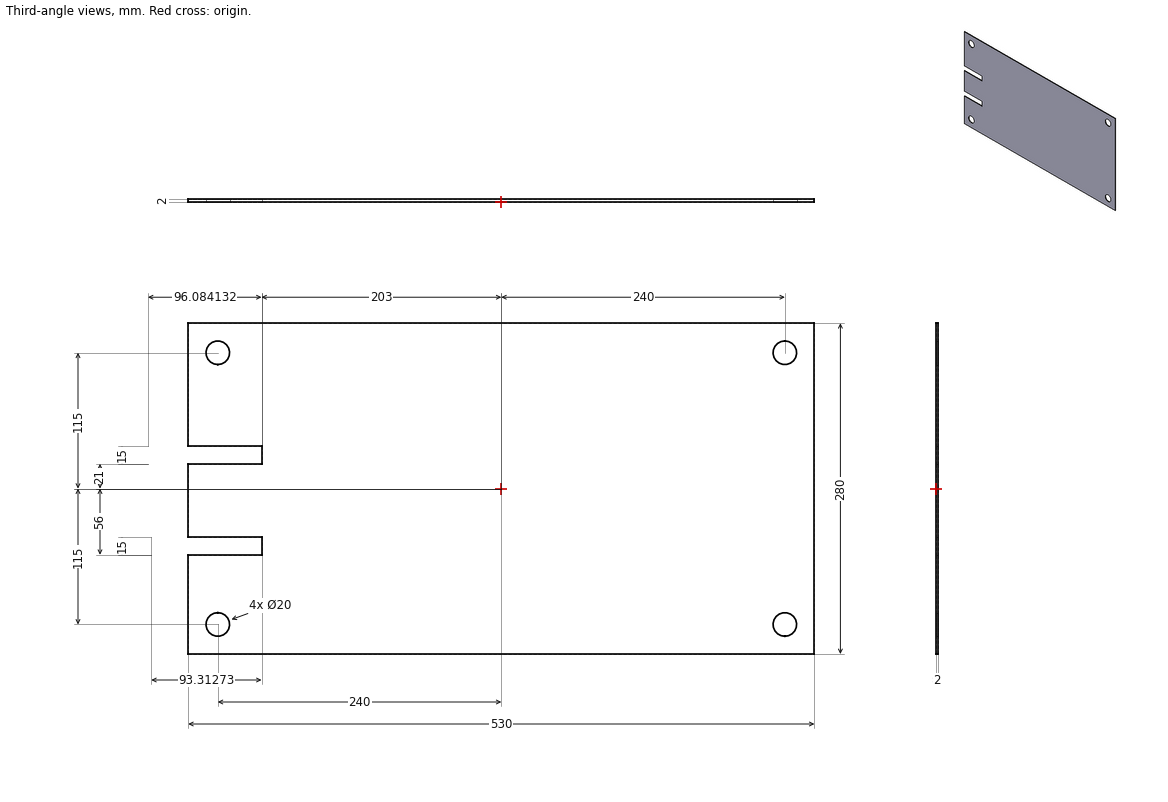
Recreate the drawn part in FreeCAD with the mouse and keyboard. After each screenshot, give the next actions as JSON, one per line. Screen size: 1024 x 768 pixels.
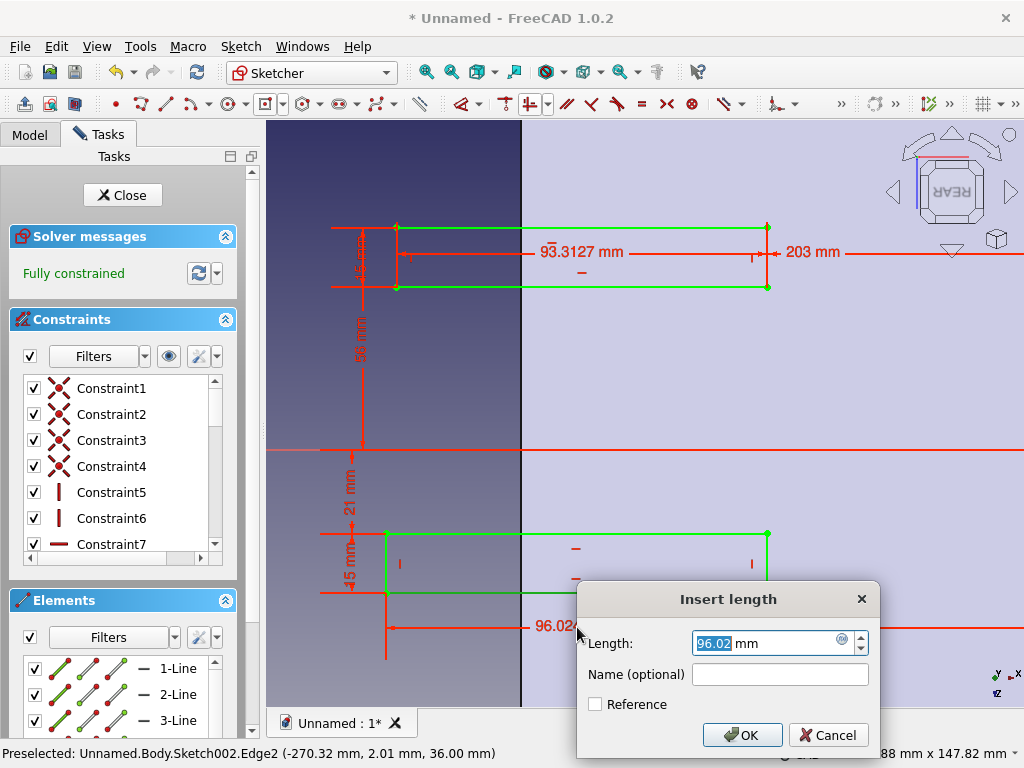
{"action": "type", "text": "96.084132"}
{"action": "key", "text": "Return"}
{"action": "key", "text": "Escape"}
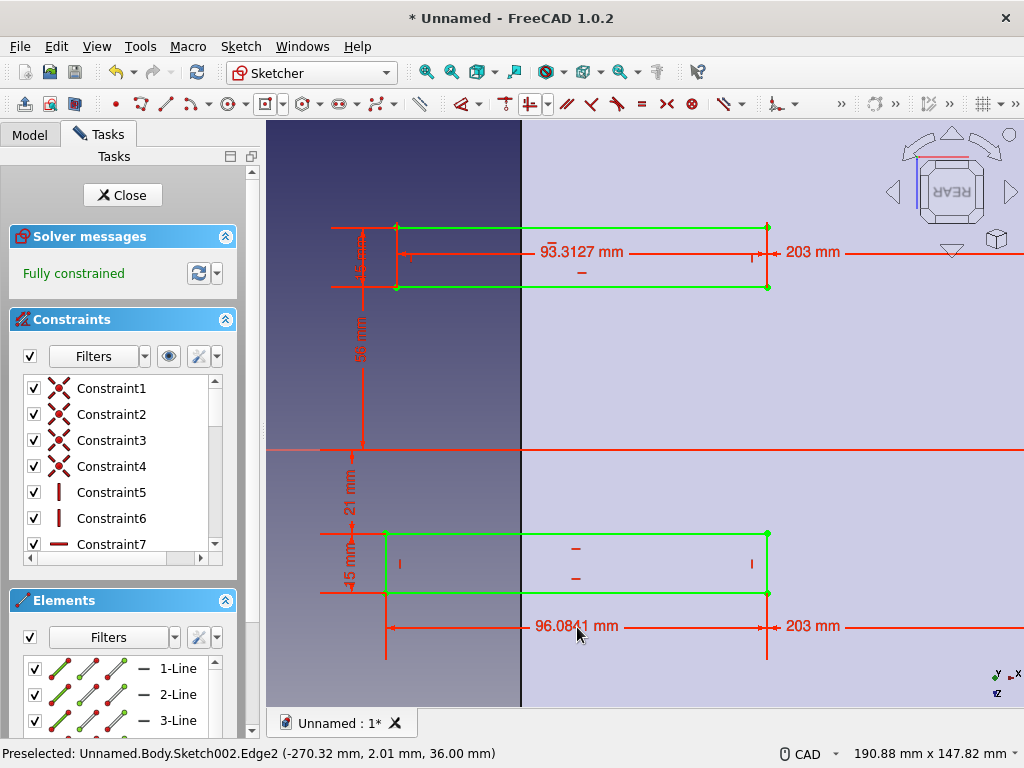
{"action": "left_click", "coordinate": [123, 195]}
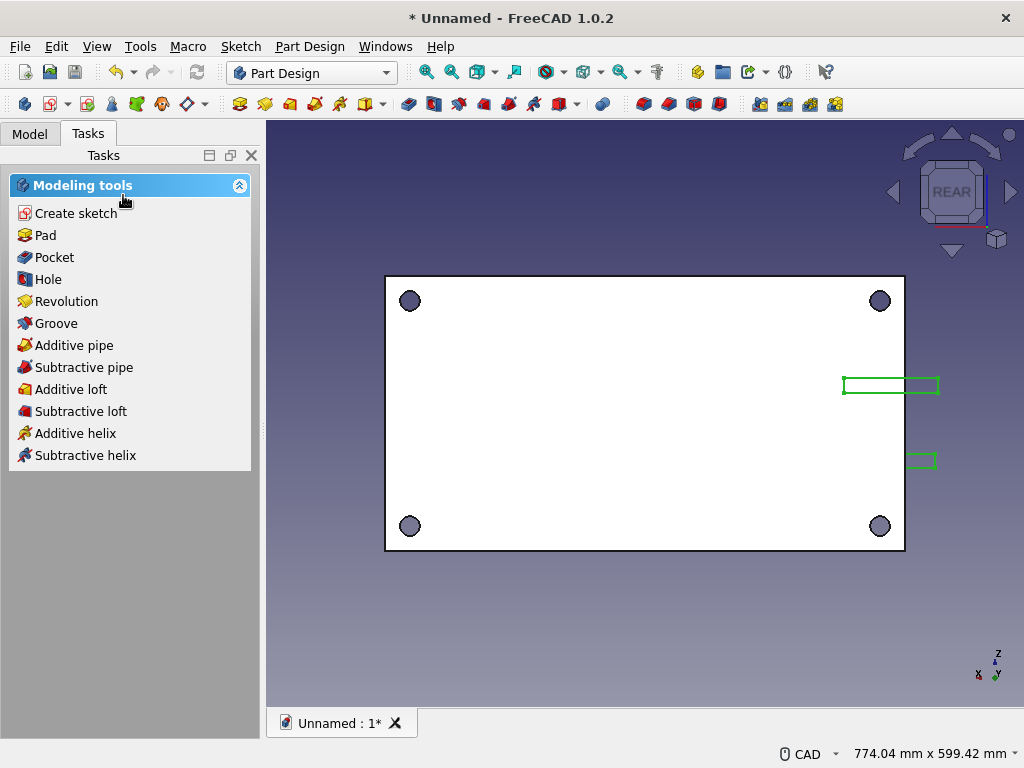
{"action": "left_click", "coordinate": [409, 104]}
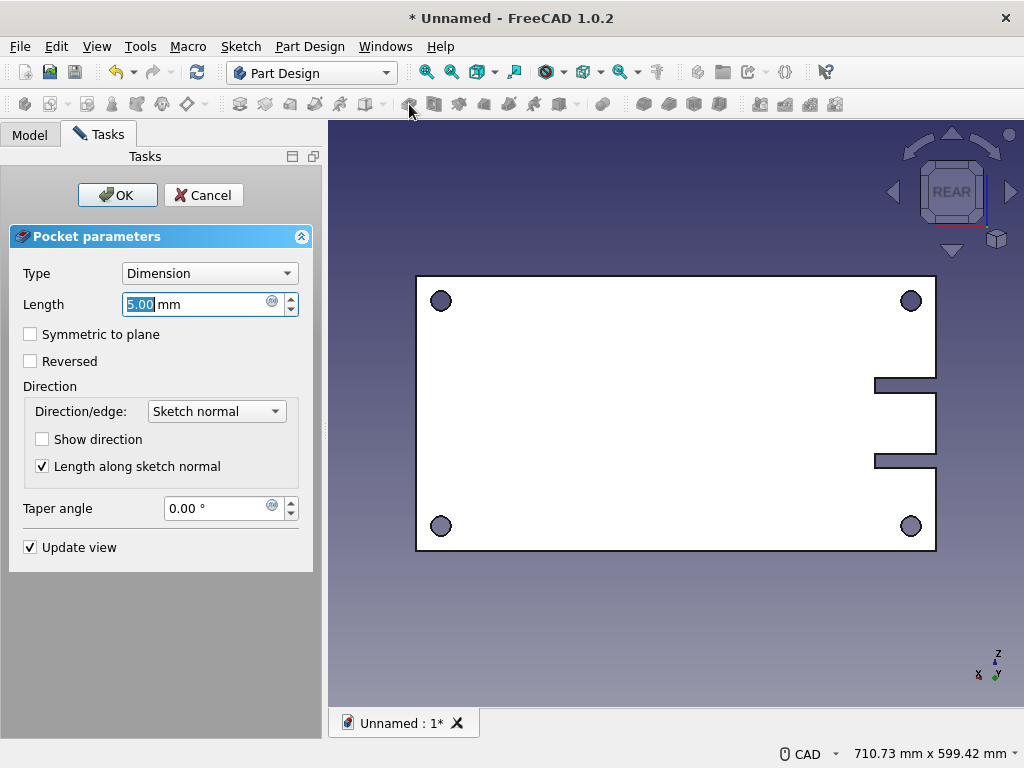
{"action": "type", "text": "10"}
{"action": "key", "text": "Tab"}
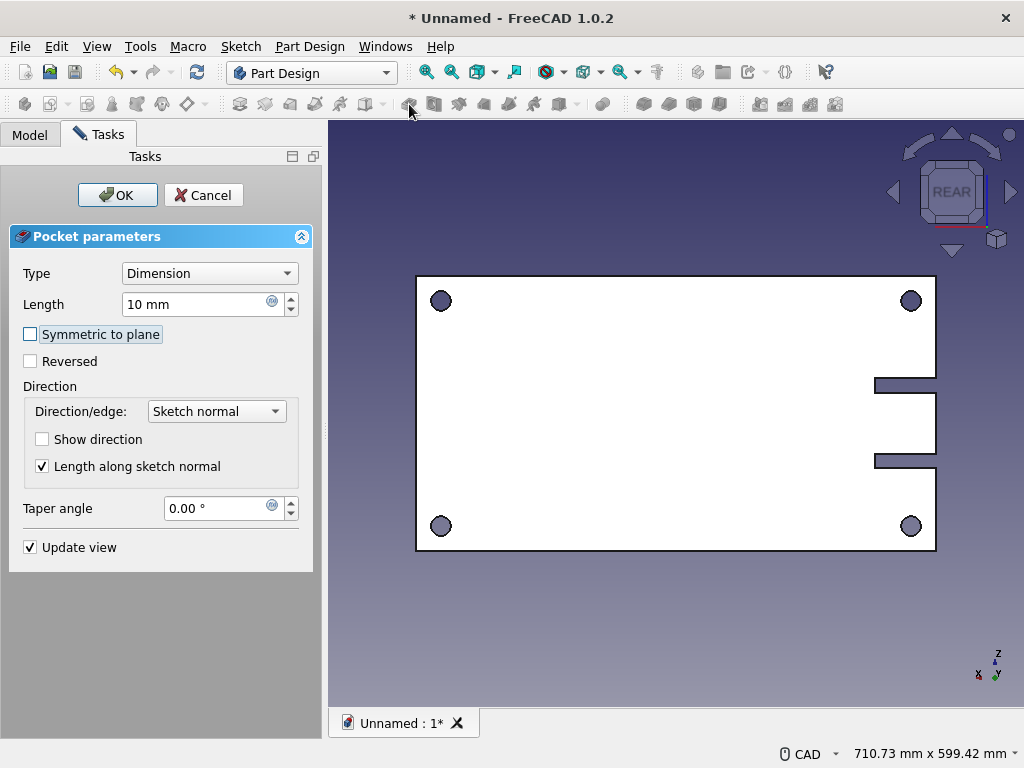
{"action": "left_click", "coordinate": [118, 195]}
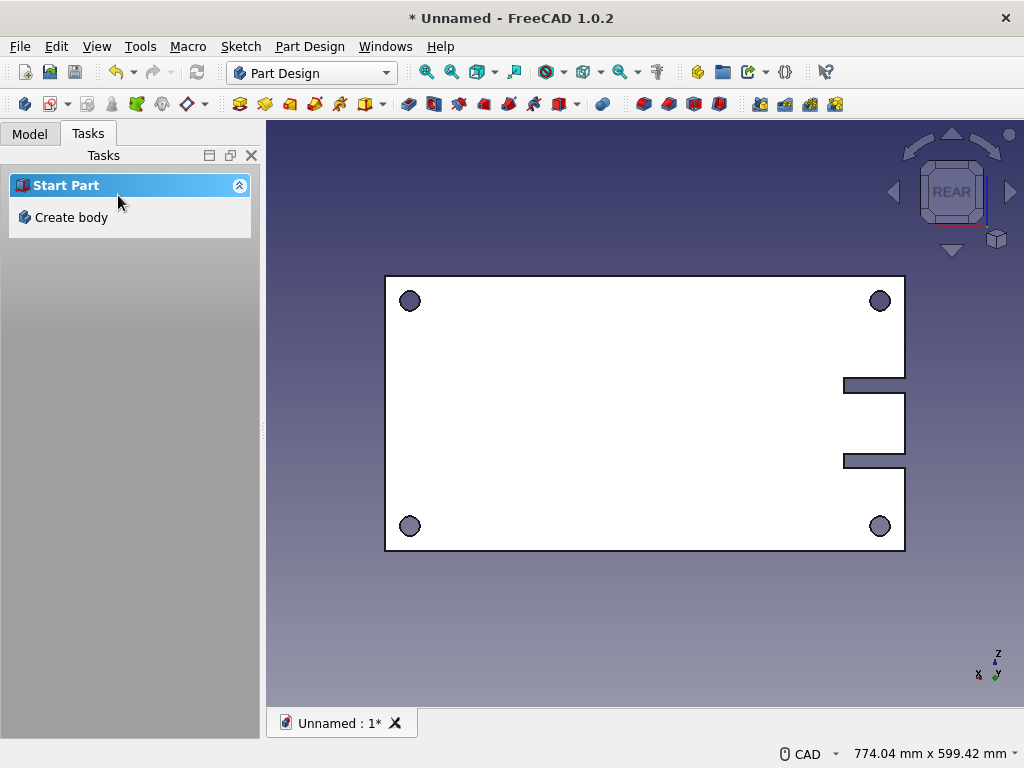
{"action": "key", "text": "0"}